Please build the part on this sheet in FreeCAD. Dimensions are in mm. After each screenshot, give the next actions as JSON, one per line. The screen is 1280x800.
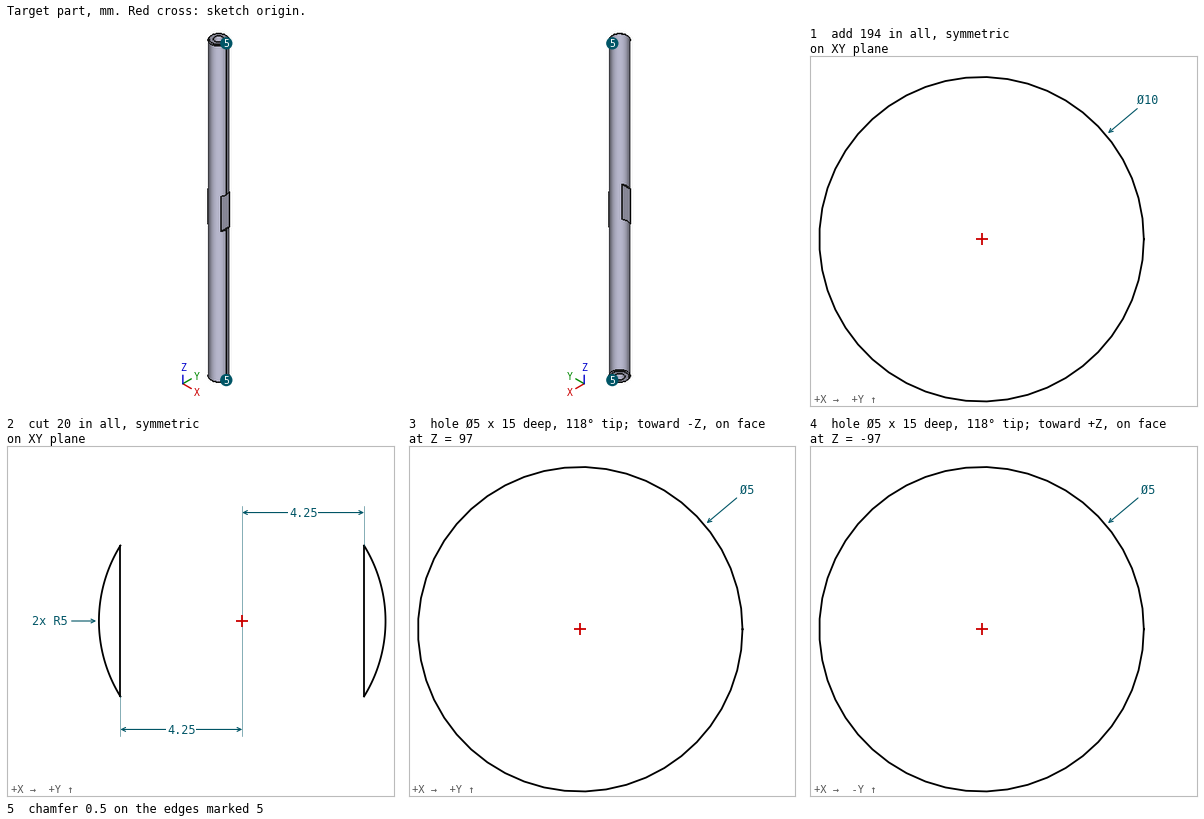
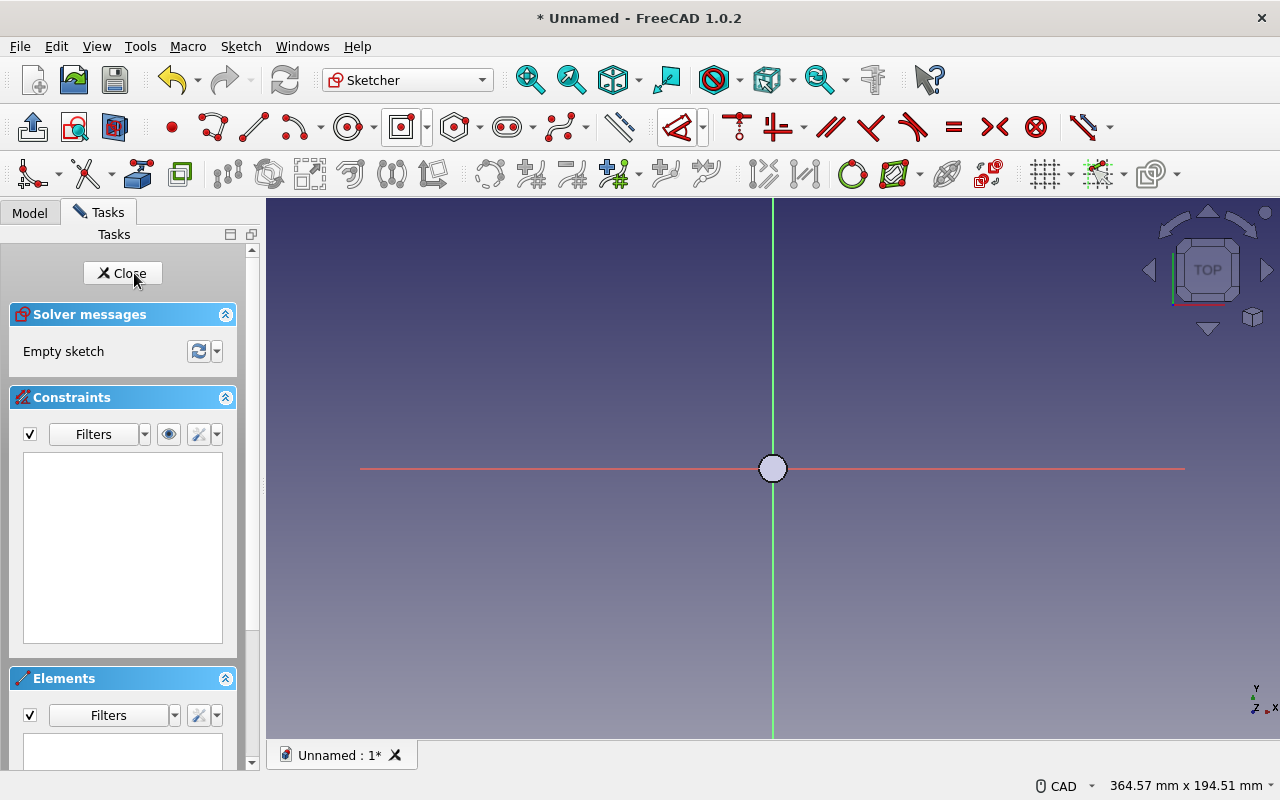
{"action": "left_click", "coordinate": [115, 128]}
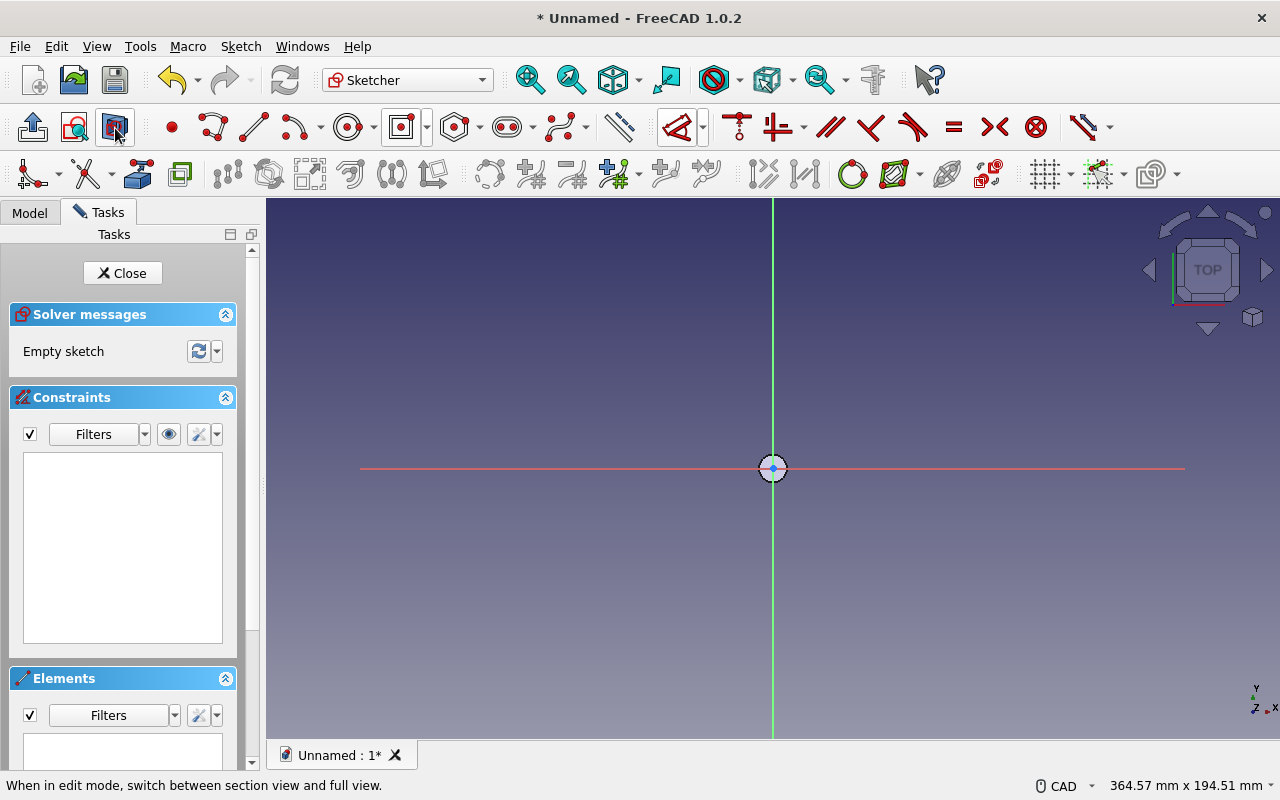
{"action": "scroll", "coordinate": [777, 468], "scroll_direction": "up", "scroll_amount": 15}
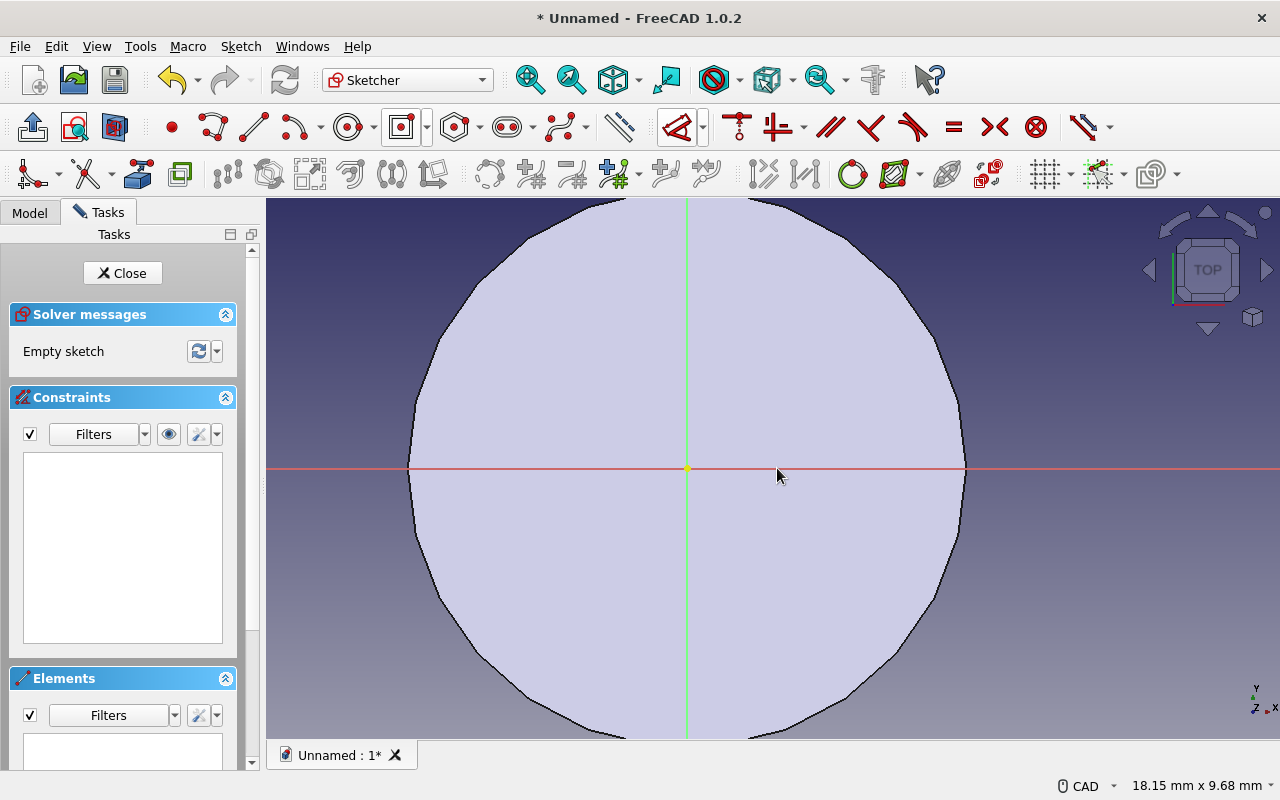
{"action": "left_click", "coordinate": [254, 128]}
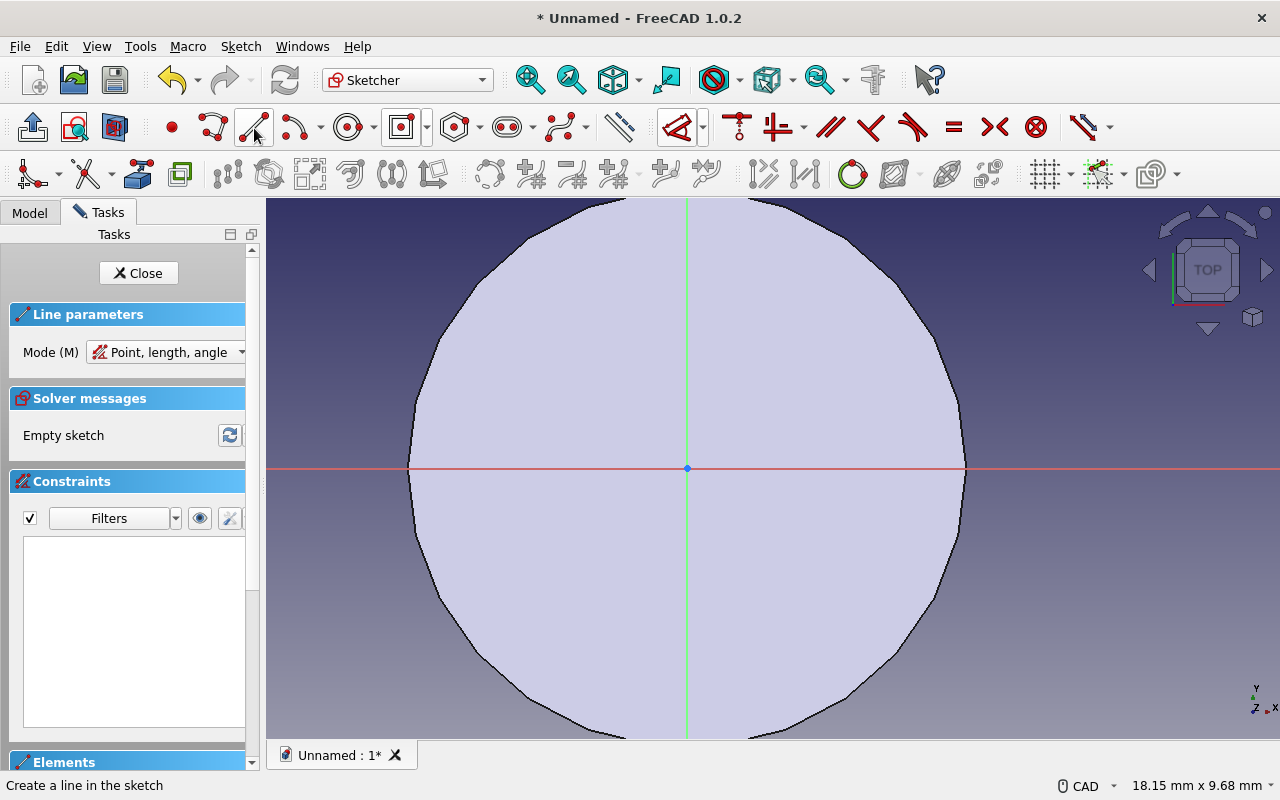
{"action": "left_click", "coordinate": [450, 616]}
{"action": "left_click", "coordinate": [450, 321]}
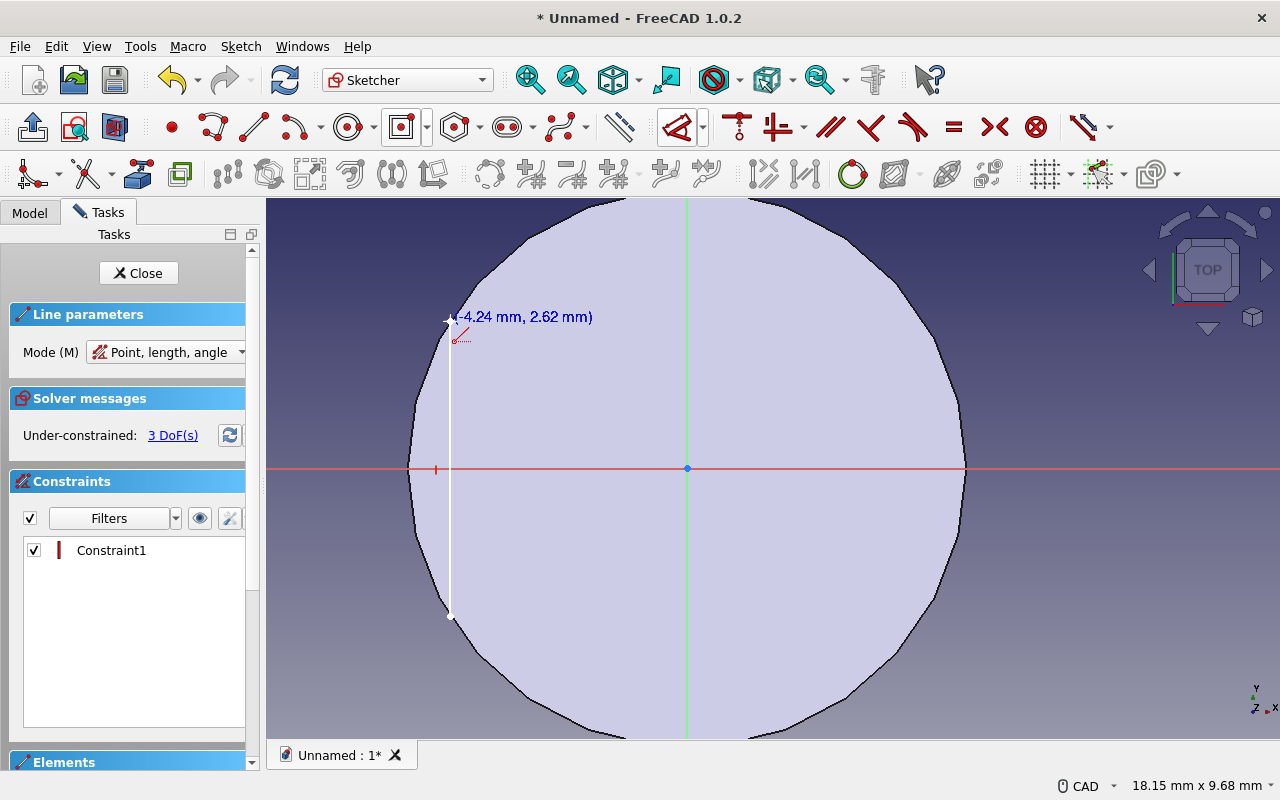
{"action": "key", "text": "g 3 a"}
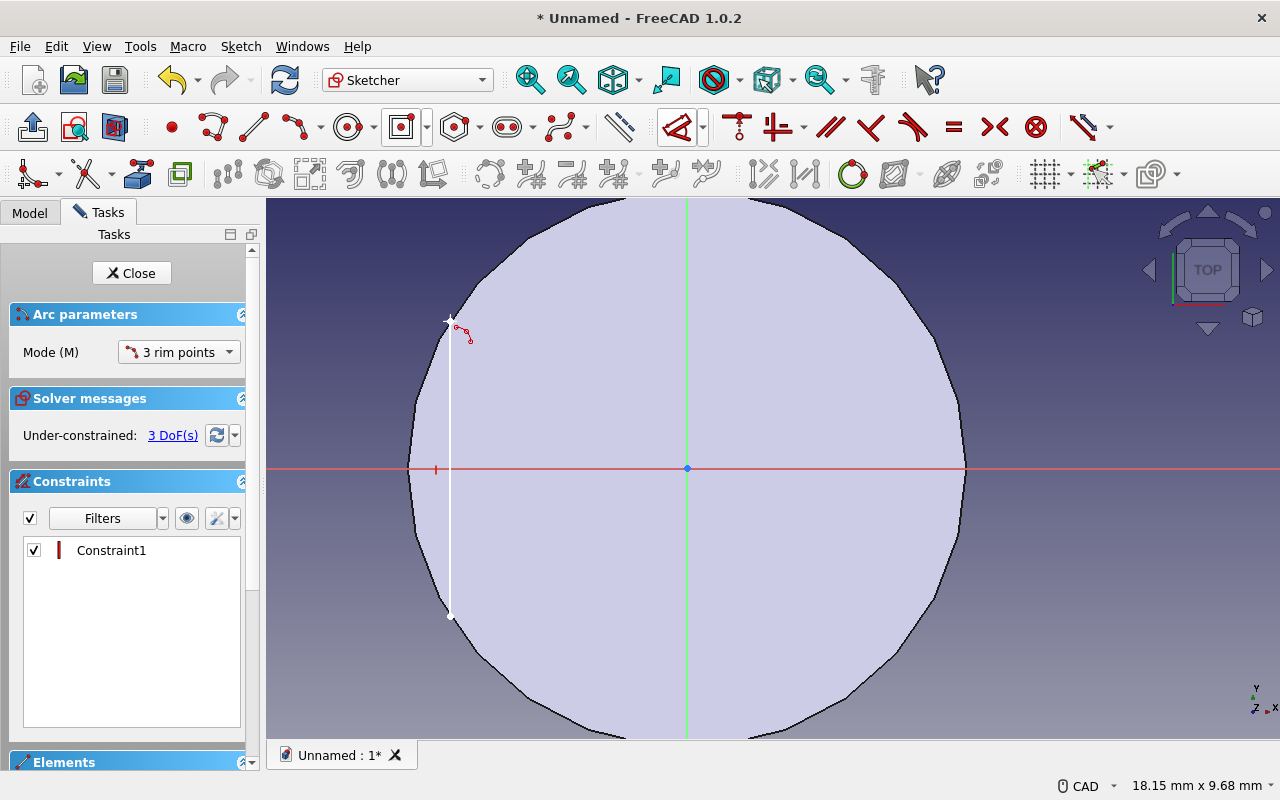
{"action": "left_click", "coordinate": [450, 322]}
{"action": "left_click", "coordinate": [450, 617]}
{"action": "left_click", "coordinate": [409, 438]}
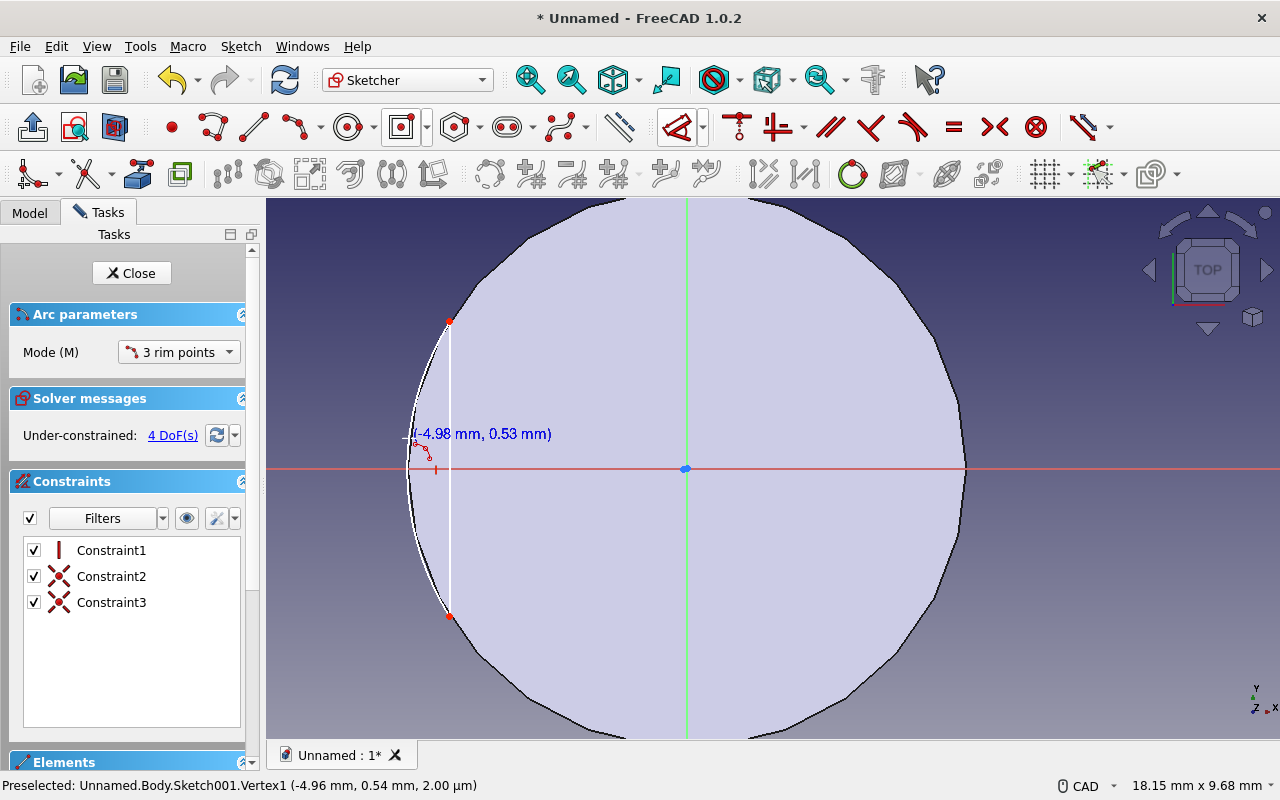
{"action": "left_click", "coordinate": [254, 128]}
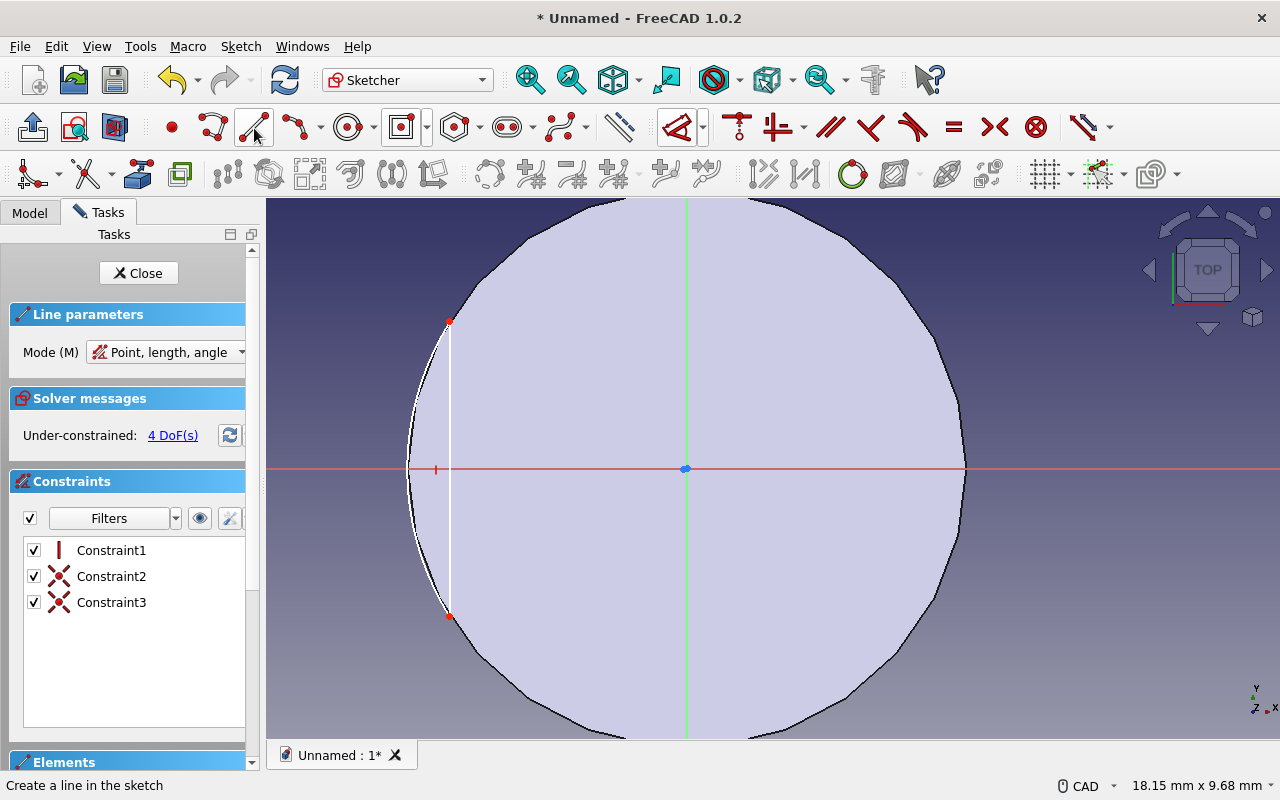
{"action": "left_click", "coordinate": [924, 321]}
{"action": "left_click", "coordinate": [924, 616]}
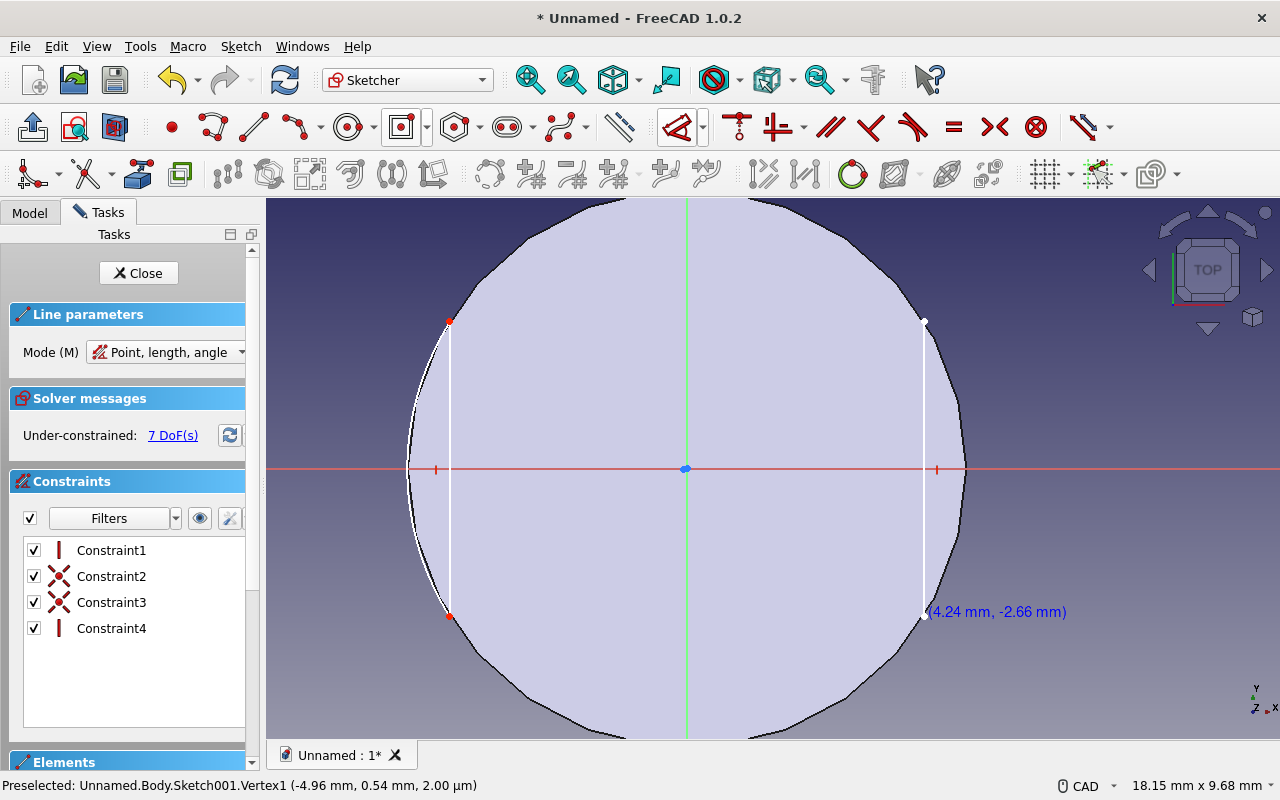
{"action": "left_click", "coordinate": [294, 128]}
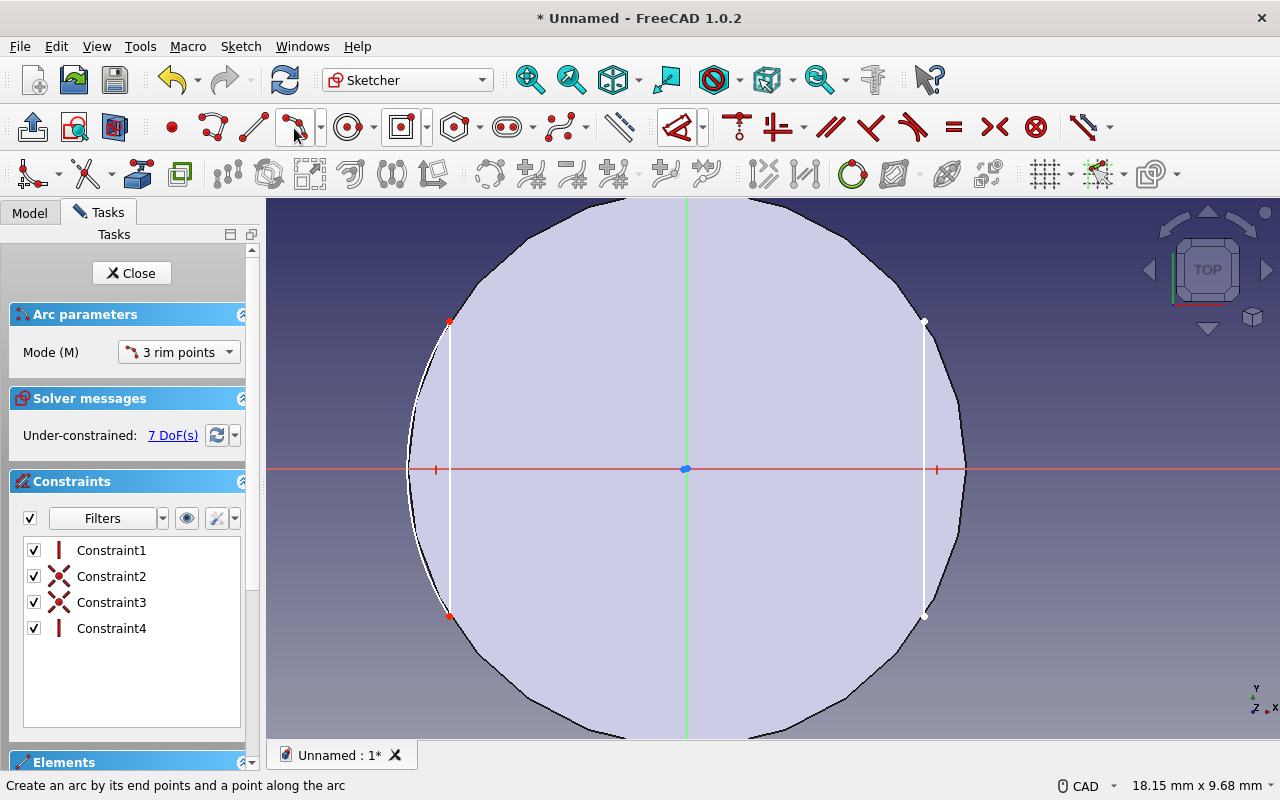
{"action": "left_click", "coordinate": [924, 617]}
{"action": "left_click", "coordinate": [924, 322]}
{"action": "left_click", "coordinate": [965, 499]}
{"action": "key", "text": "Escape"}